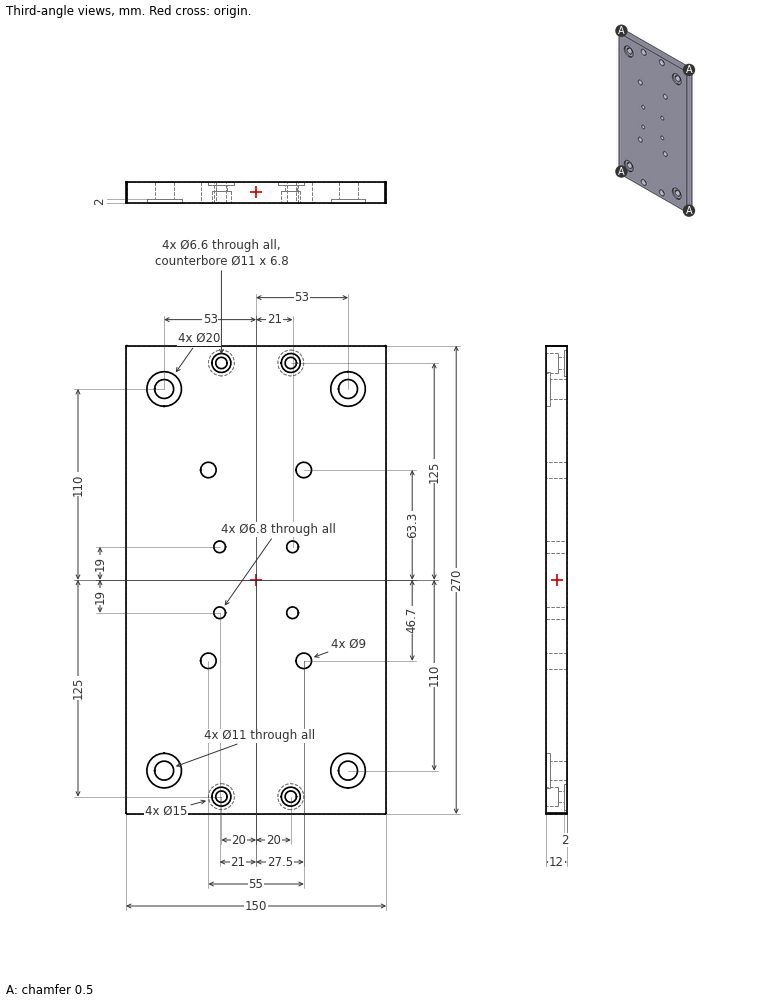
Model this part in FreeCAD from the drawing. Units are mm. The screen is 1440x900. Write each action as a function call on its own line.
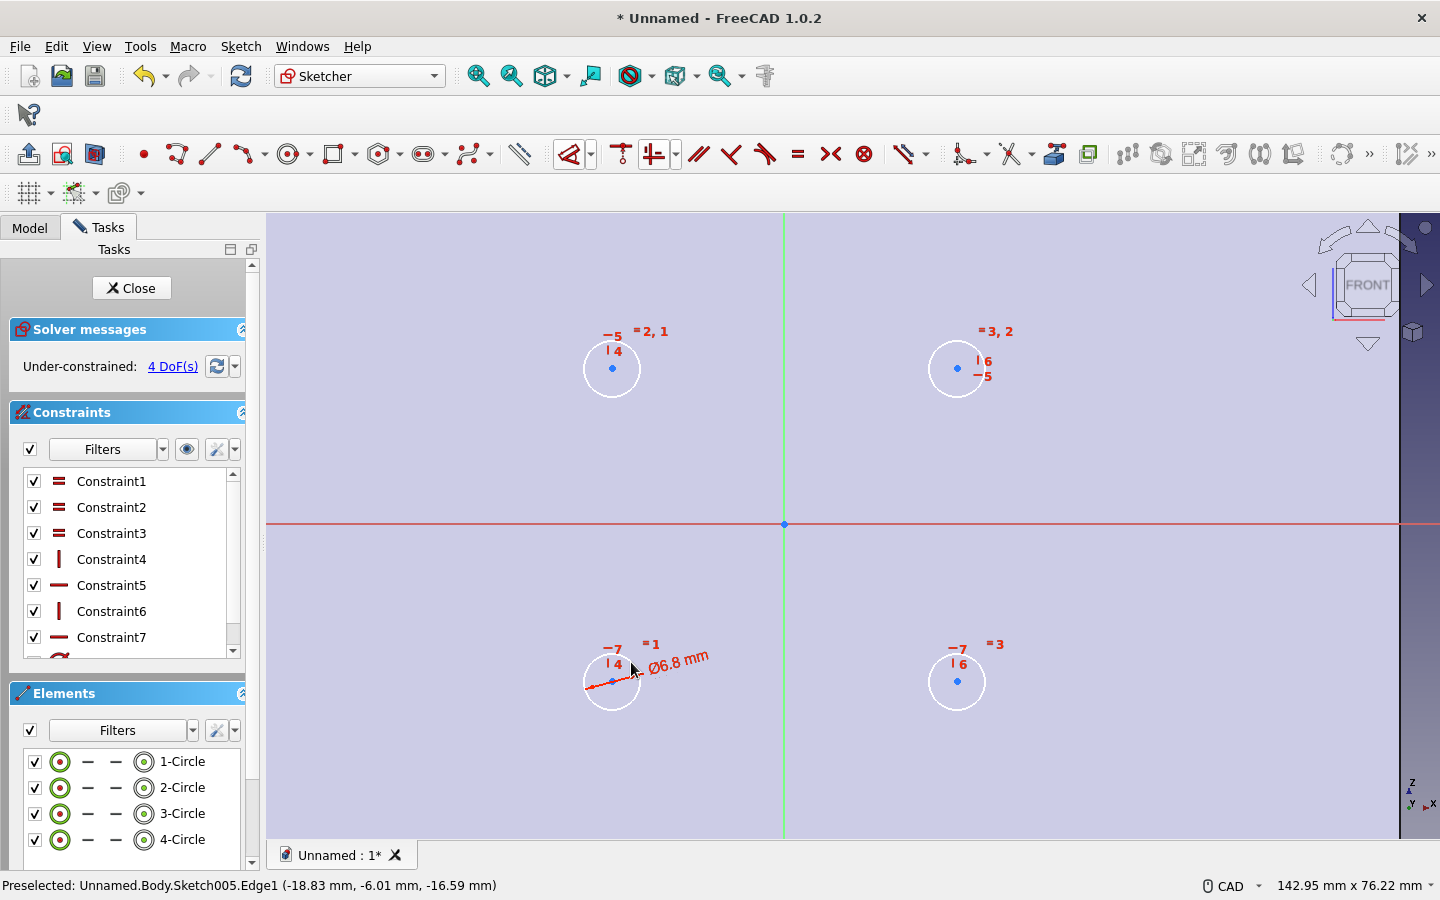
click(612, 682)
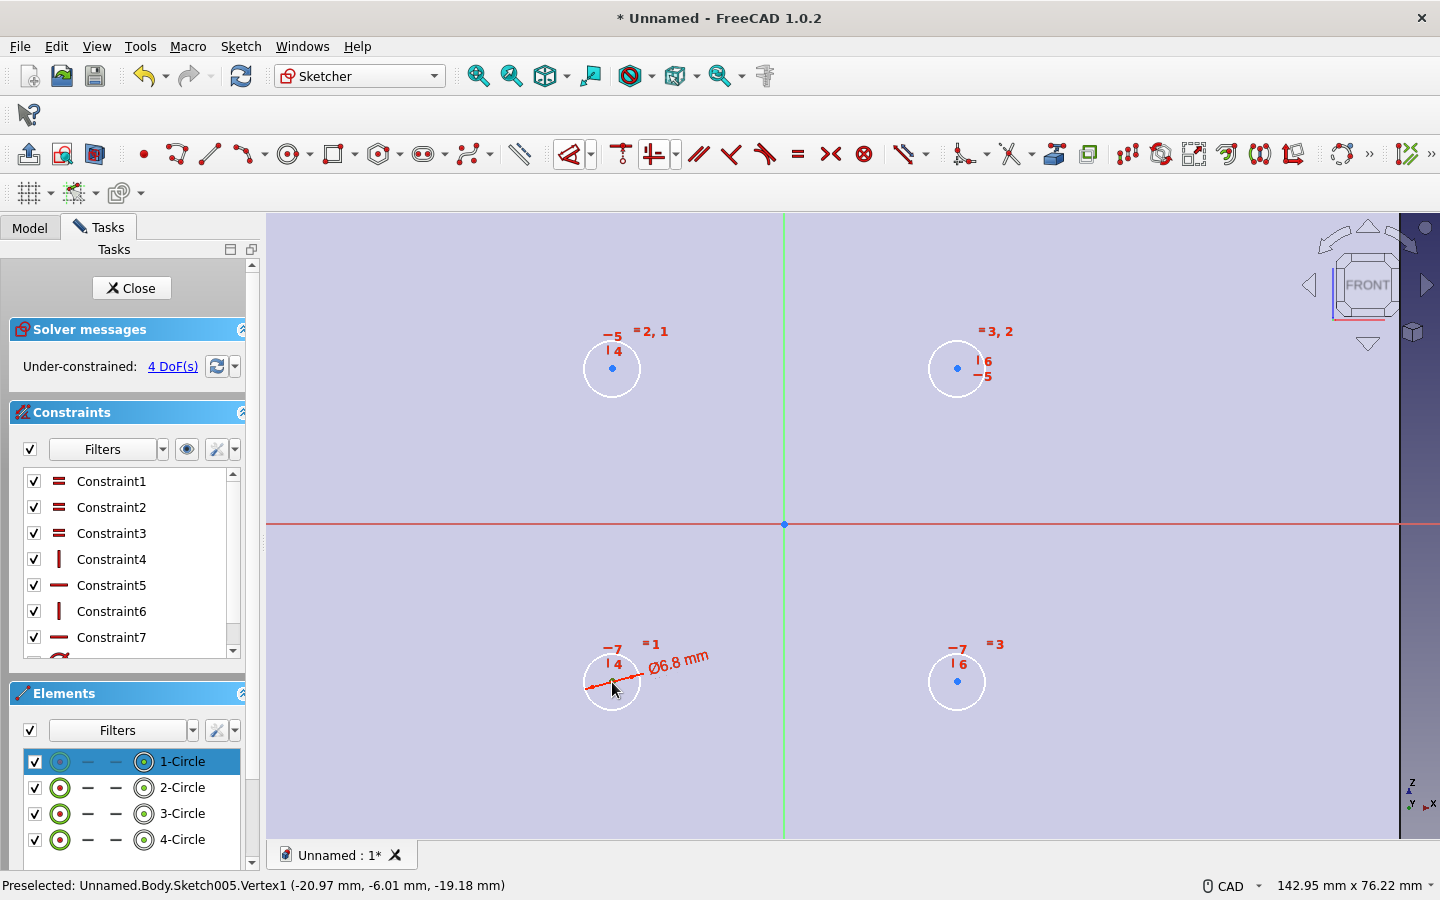
key(l)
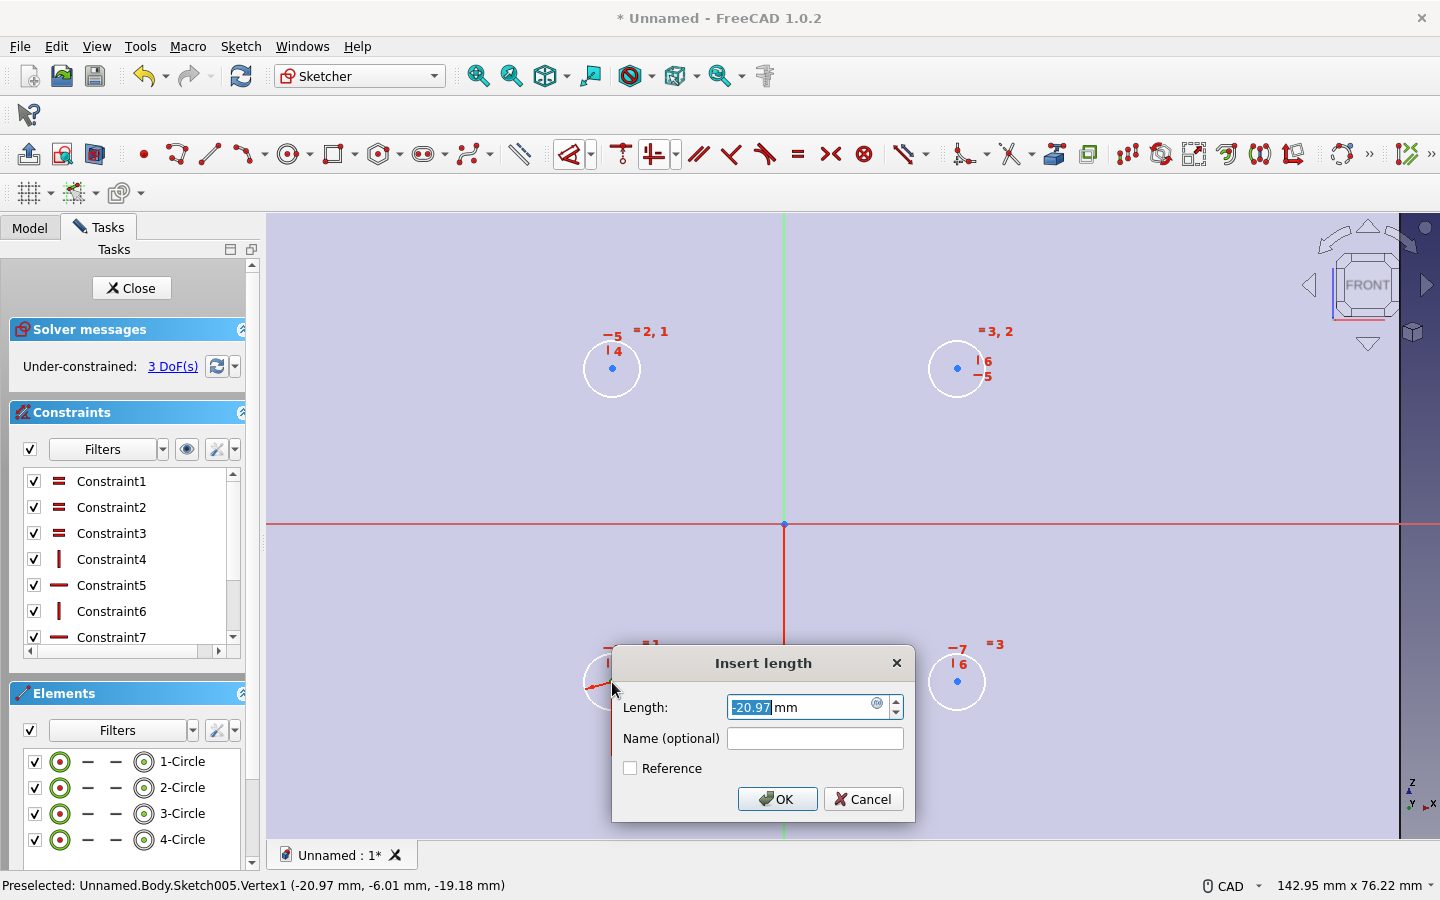
text(-21)
key(Return)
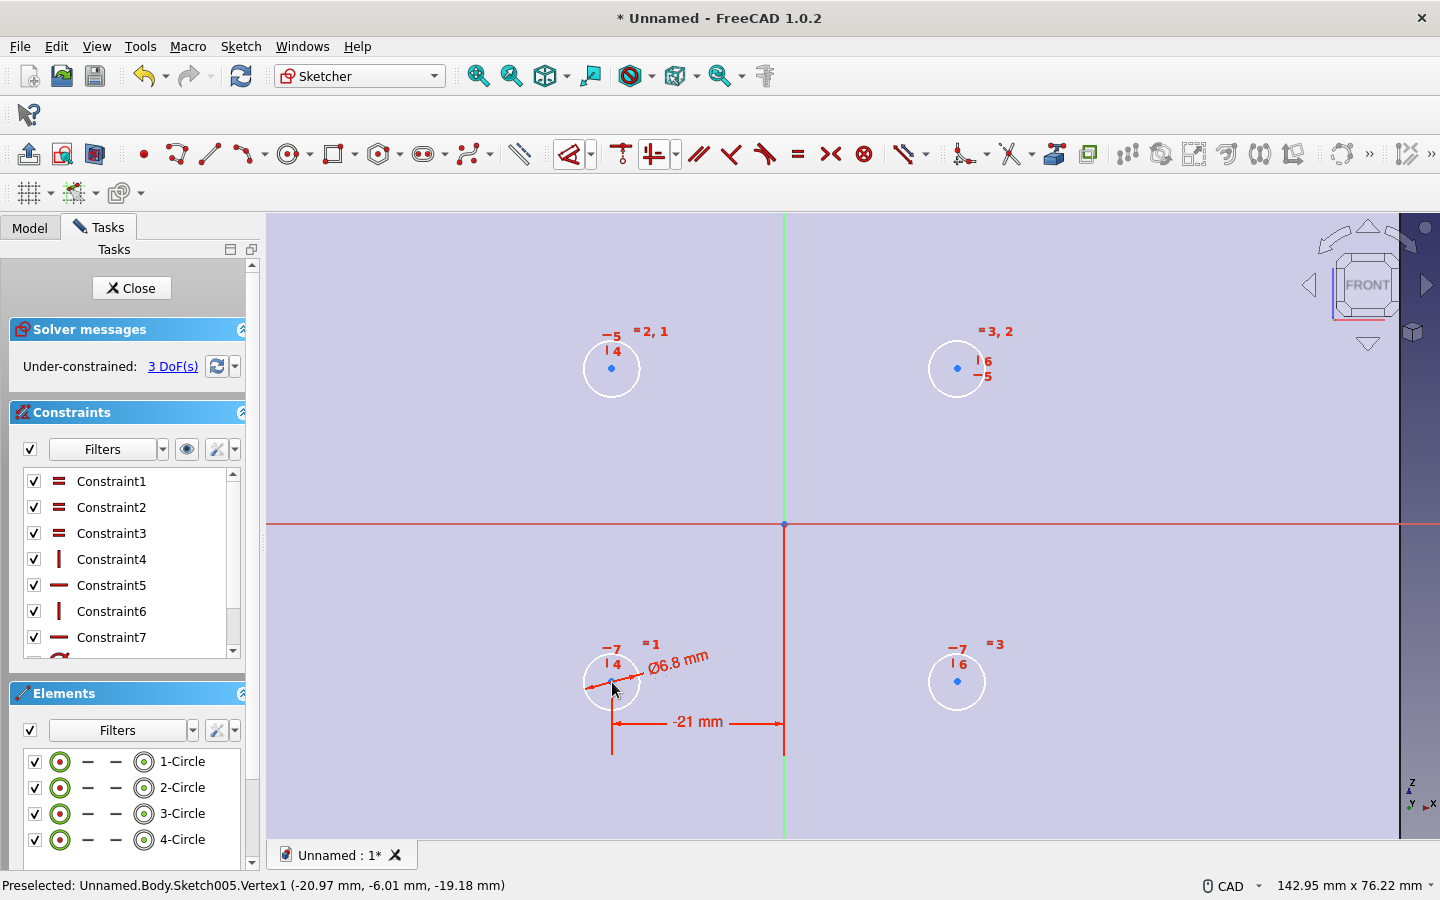
click(612, 682)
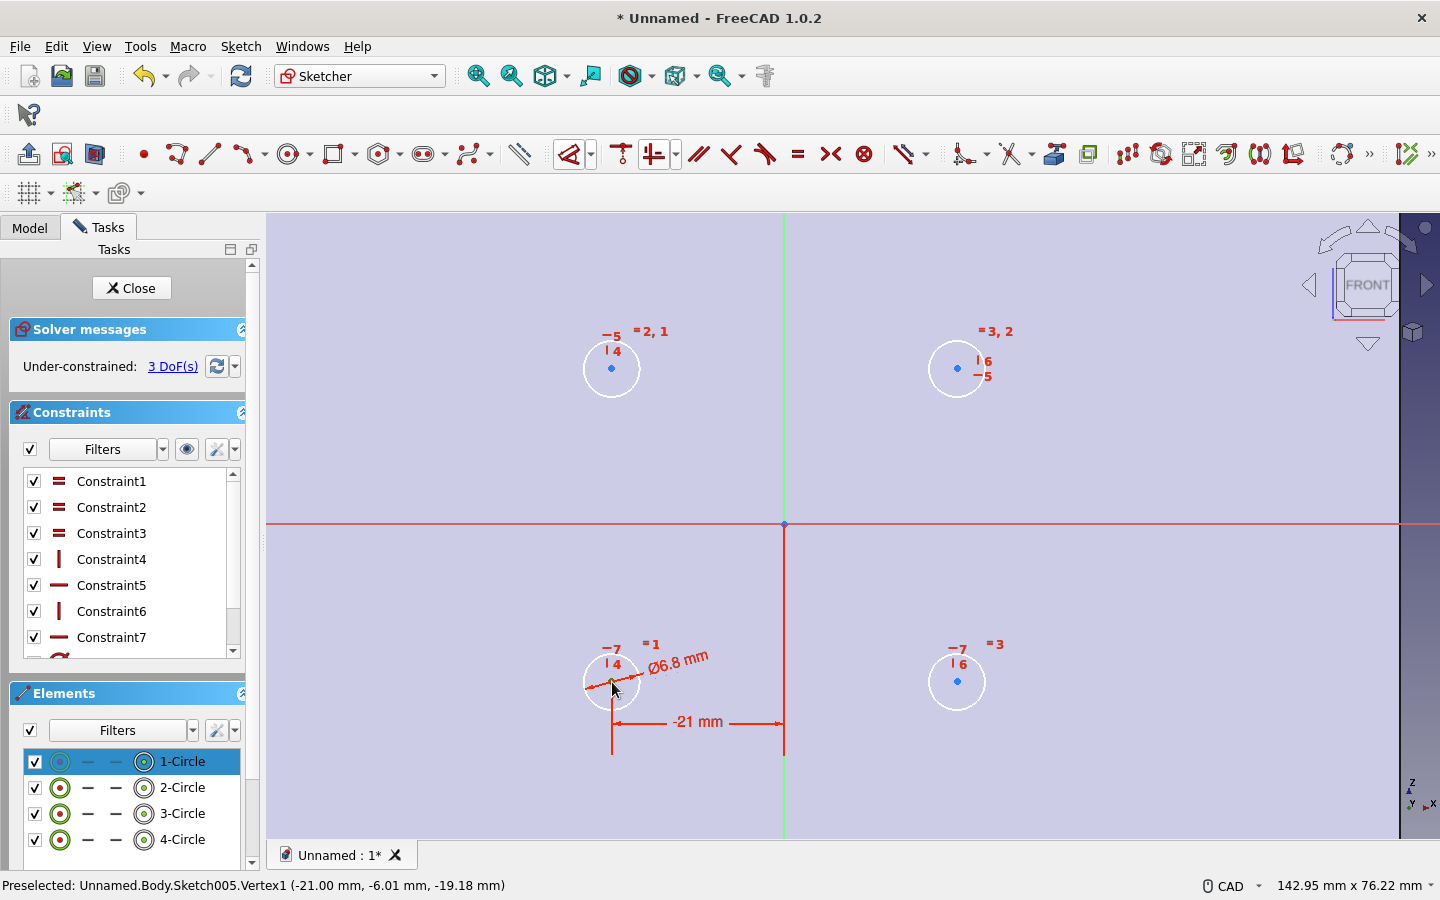
key(i)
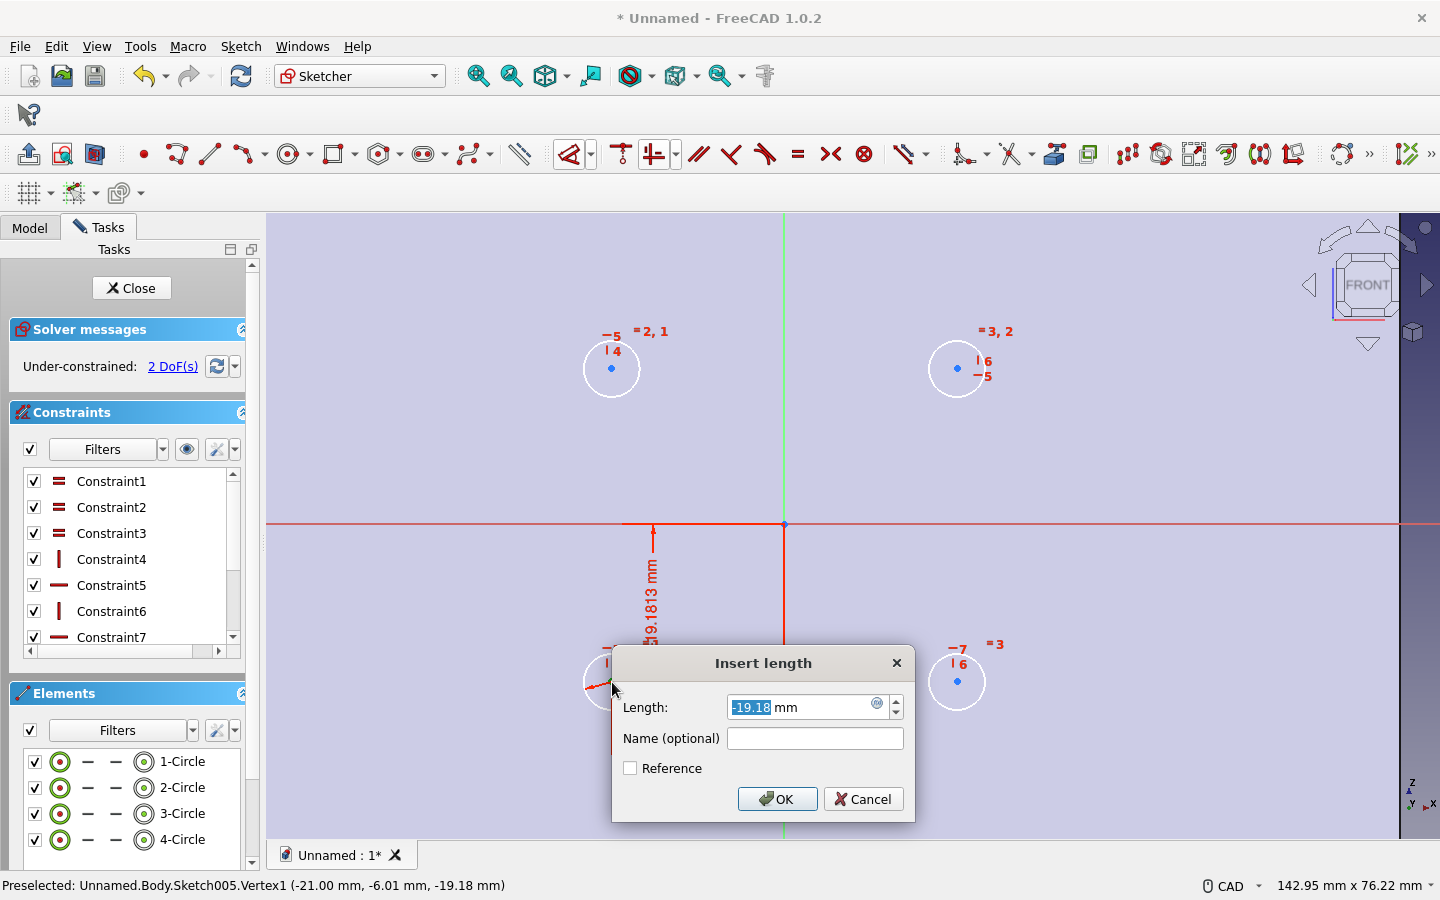
text(-19)
key(Return)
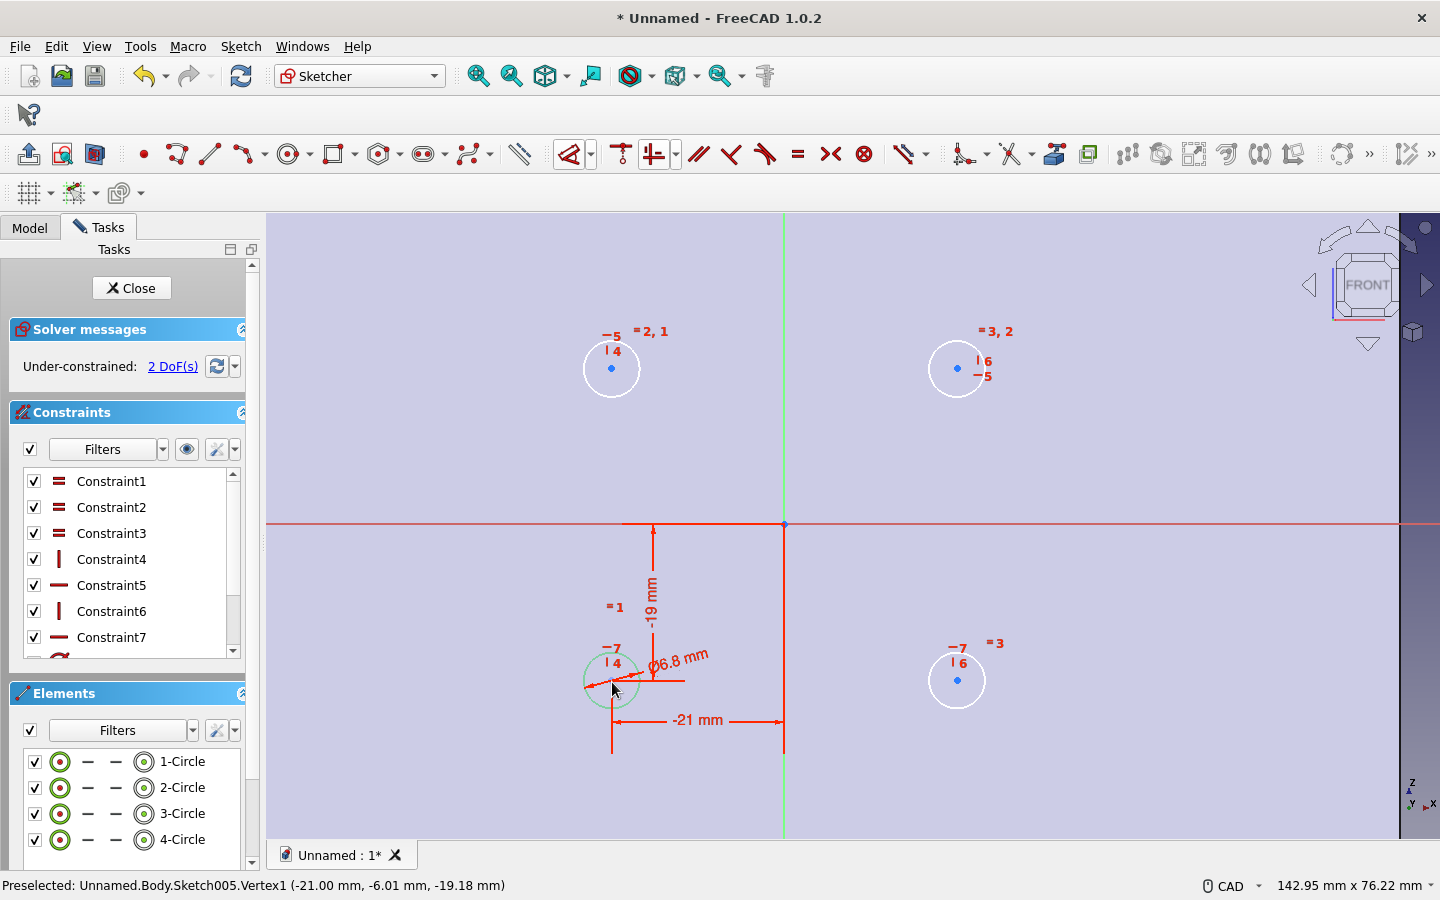
click(612, 369)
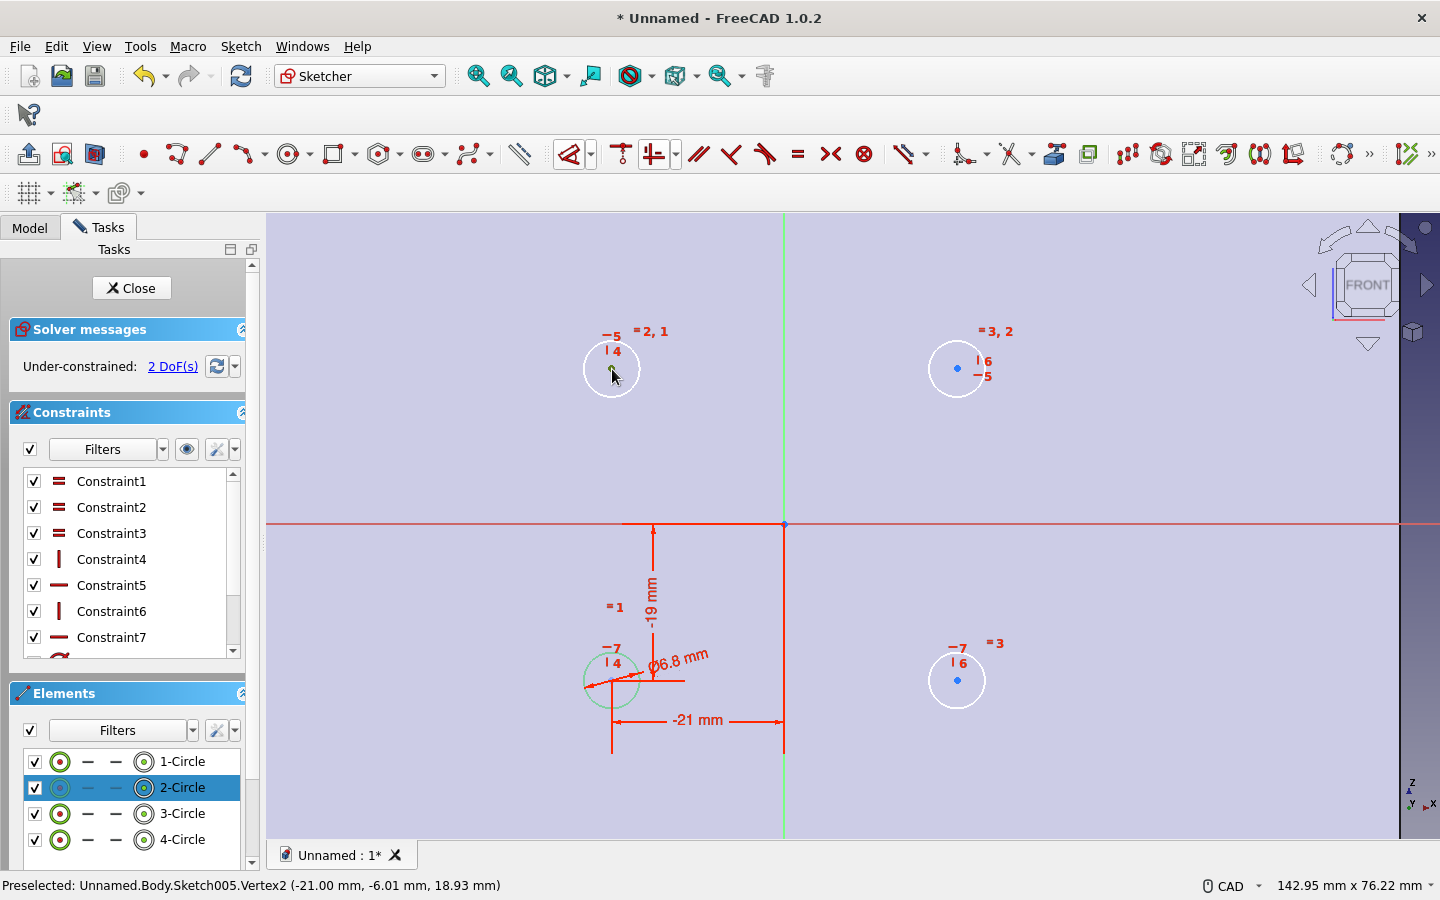
key(i)